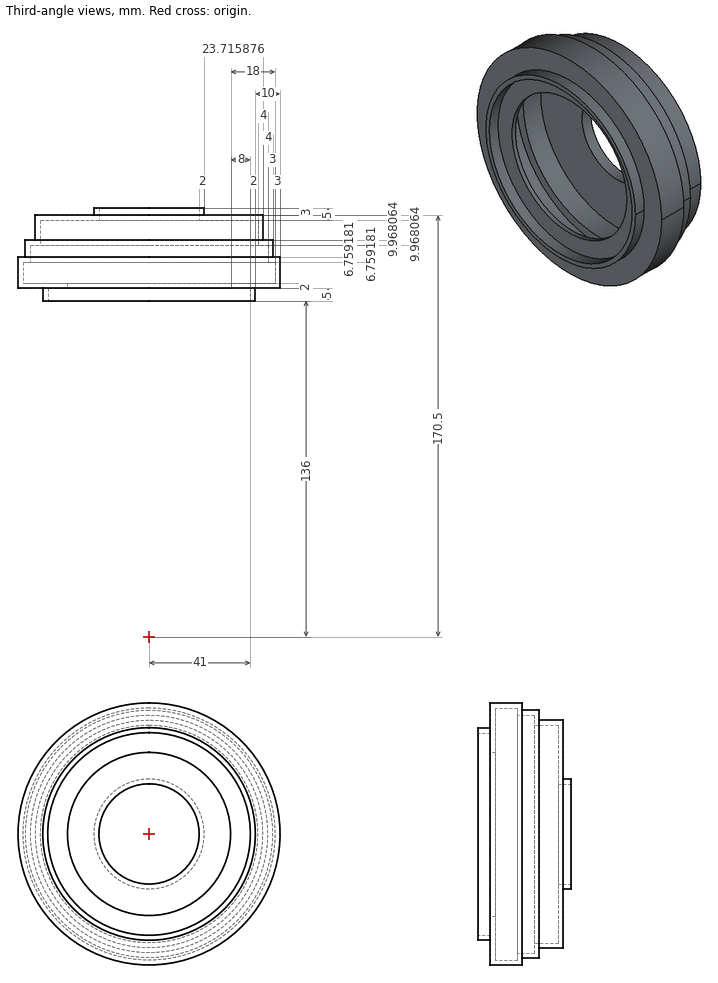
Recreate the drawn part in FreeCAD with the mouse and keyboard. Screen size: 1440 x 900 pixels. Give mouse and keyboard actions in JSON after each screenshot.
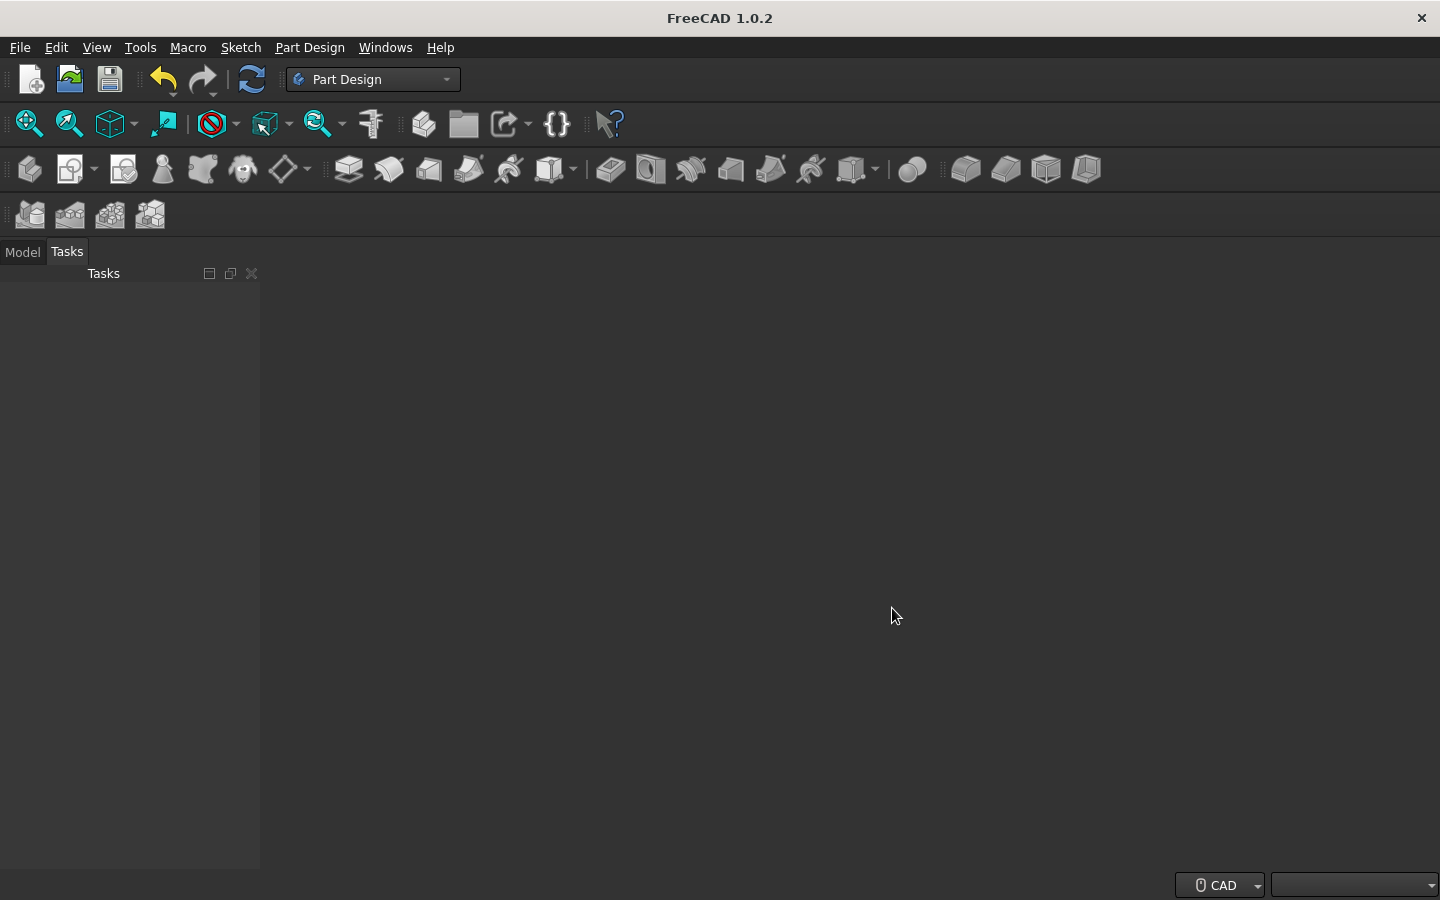
{"action": "left_click", "coordinate": [30, 80]}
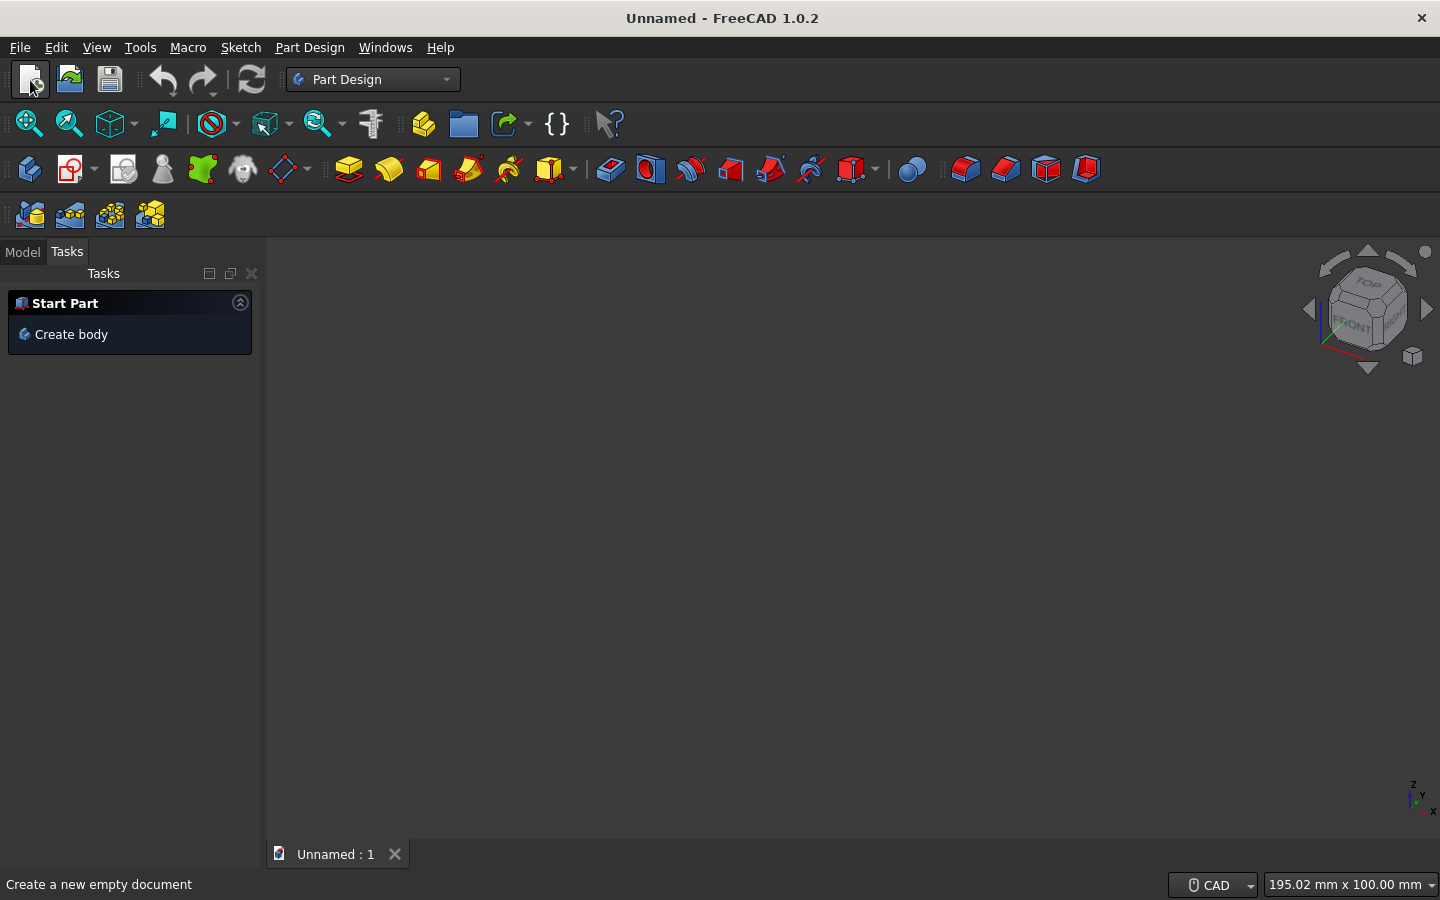
{"action": "left_click", "coordinate": [70, 170]}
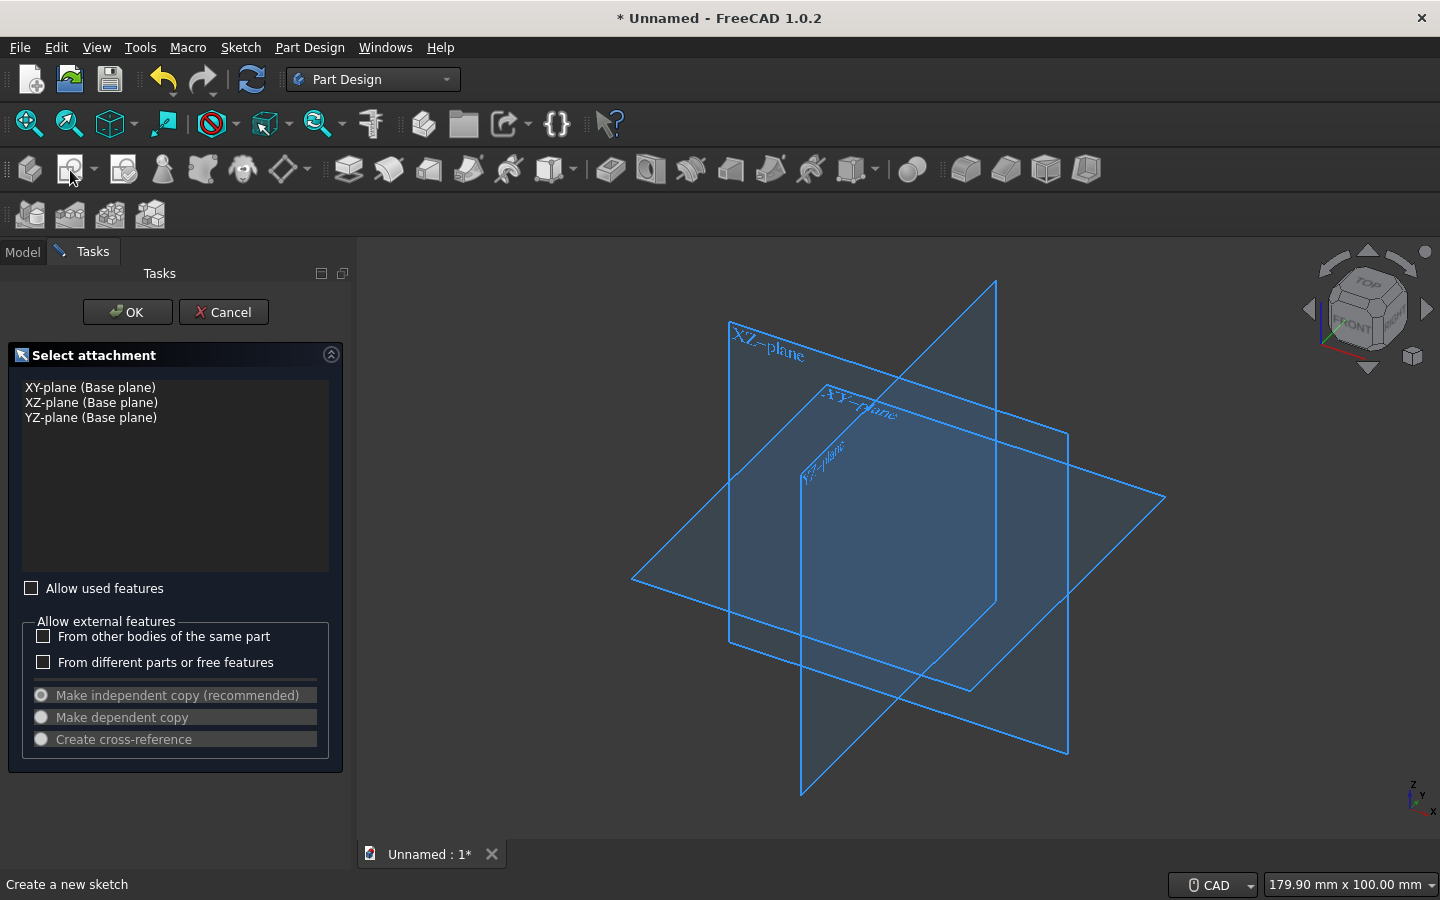
{"action": "left_click", "coordinate": [82, 388]}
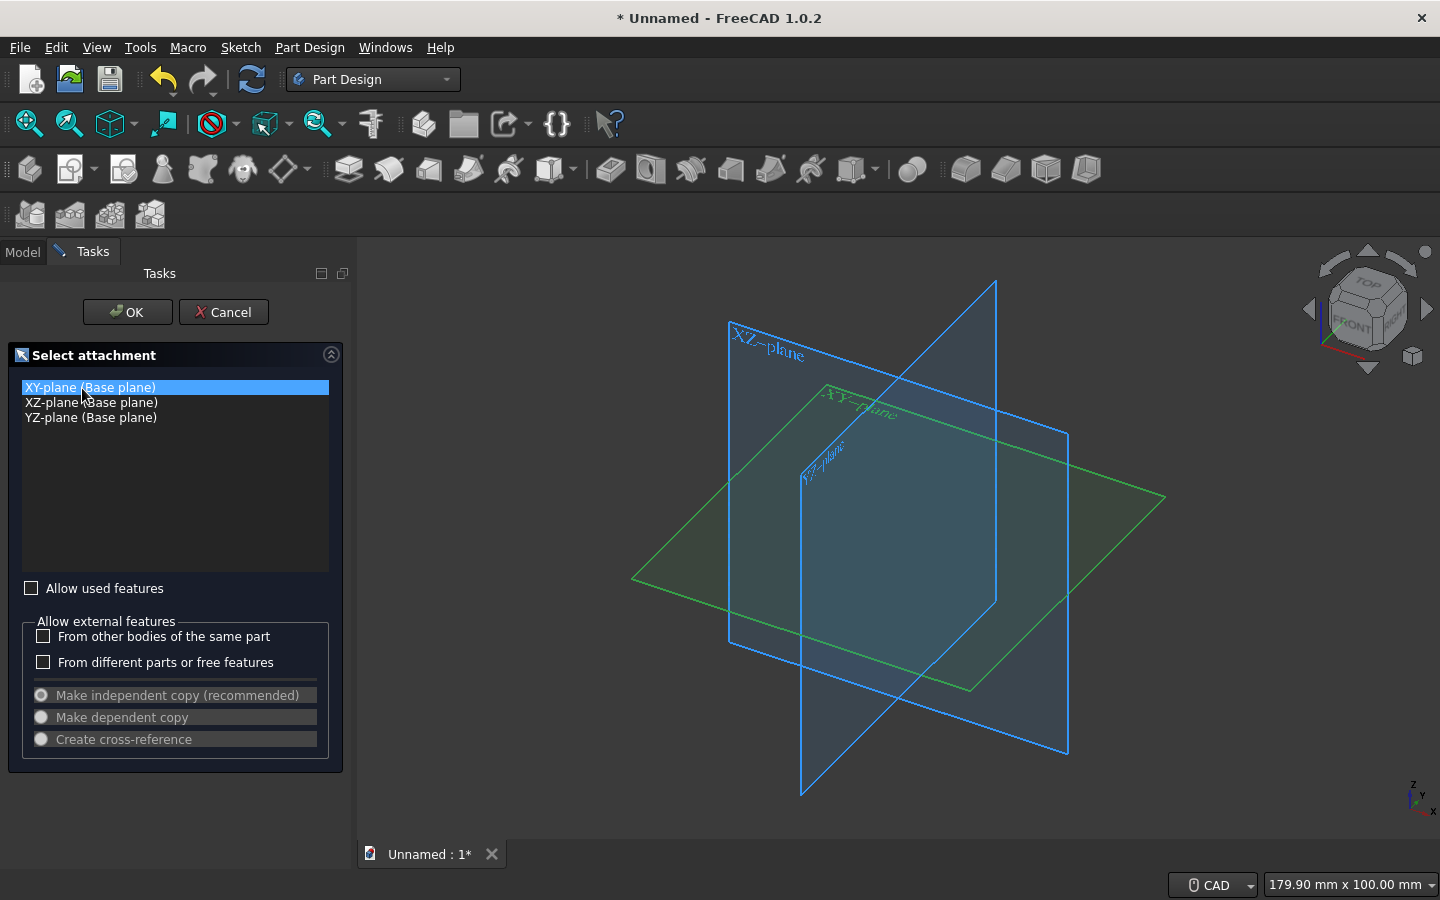
{"action": "left_click", "coordinate": [128, 312]}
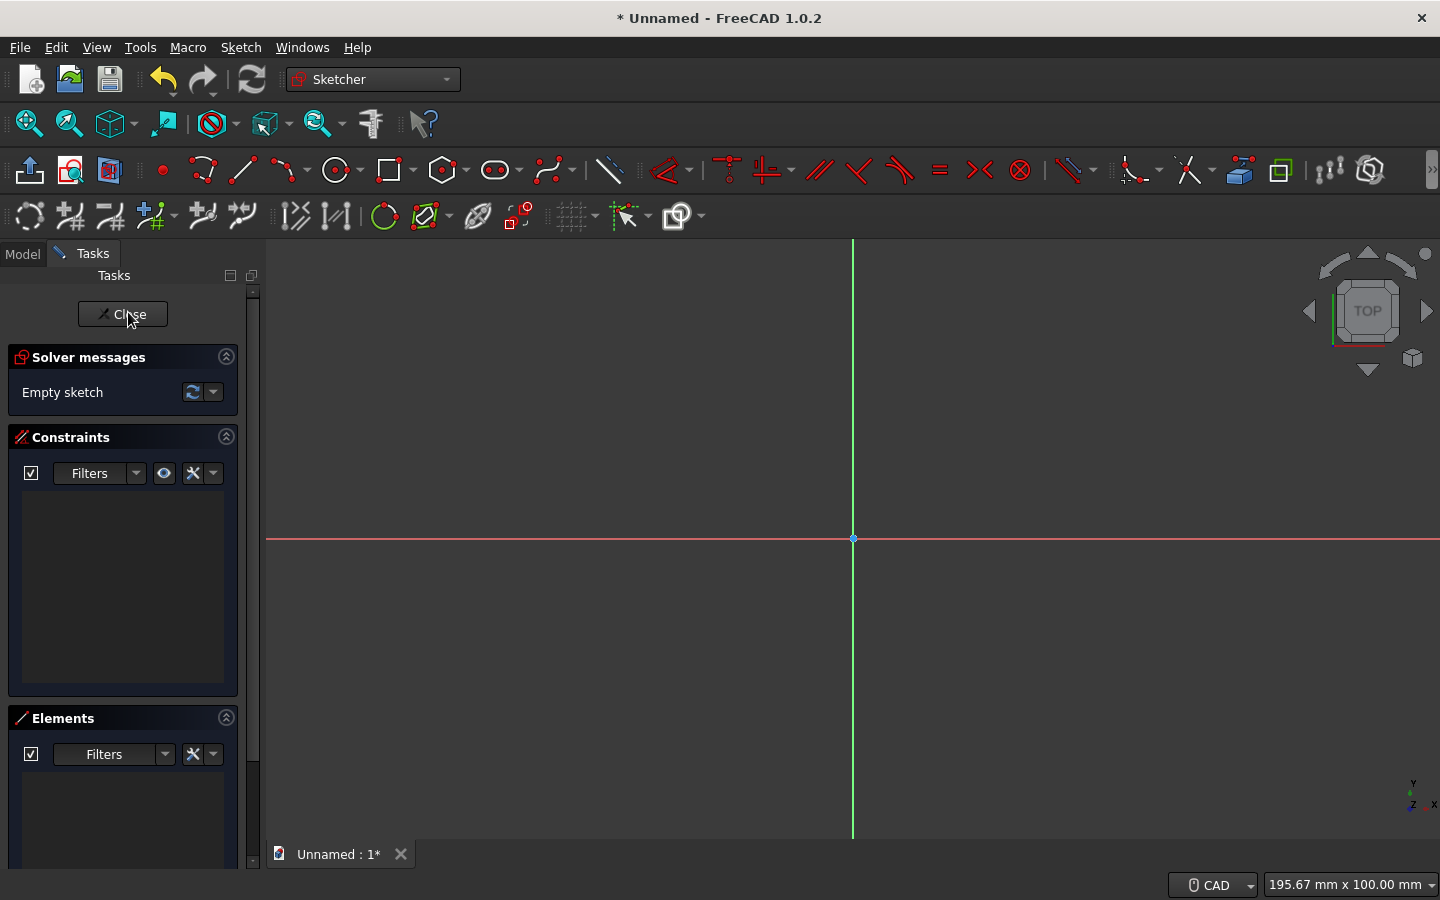
{"action": "scroll", "coordinate": [784, 539], "scroll_direction": "down", "scroll_amount": 5}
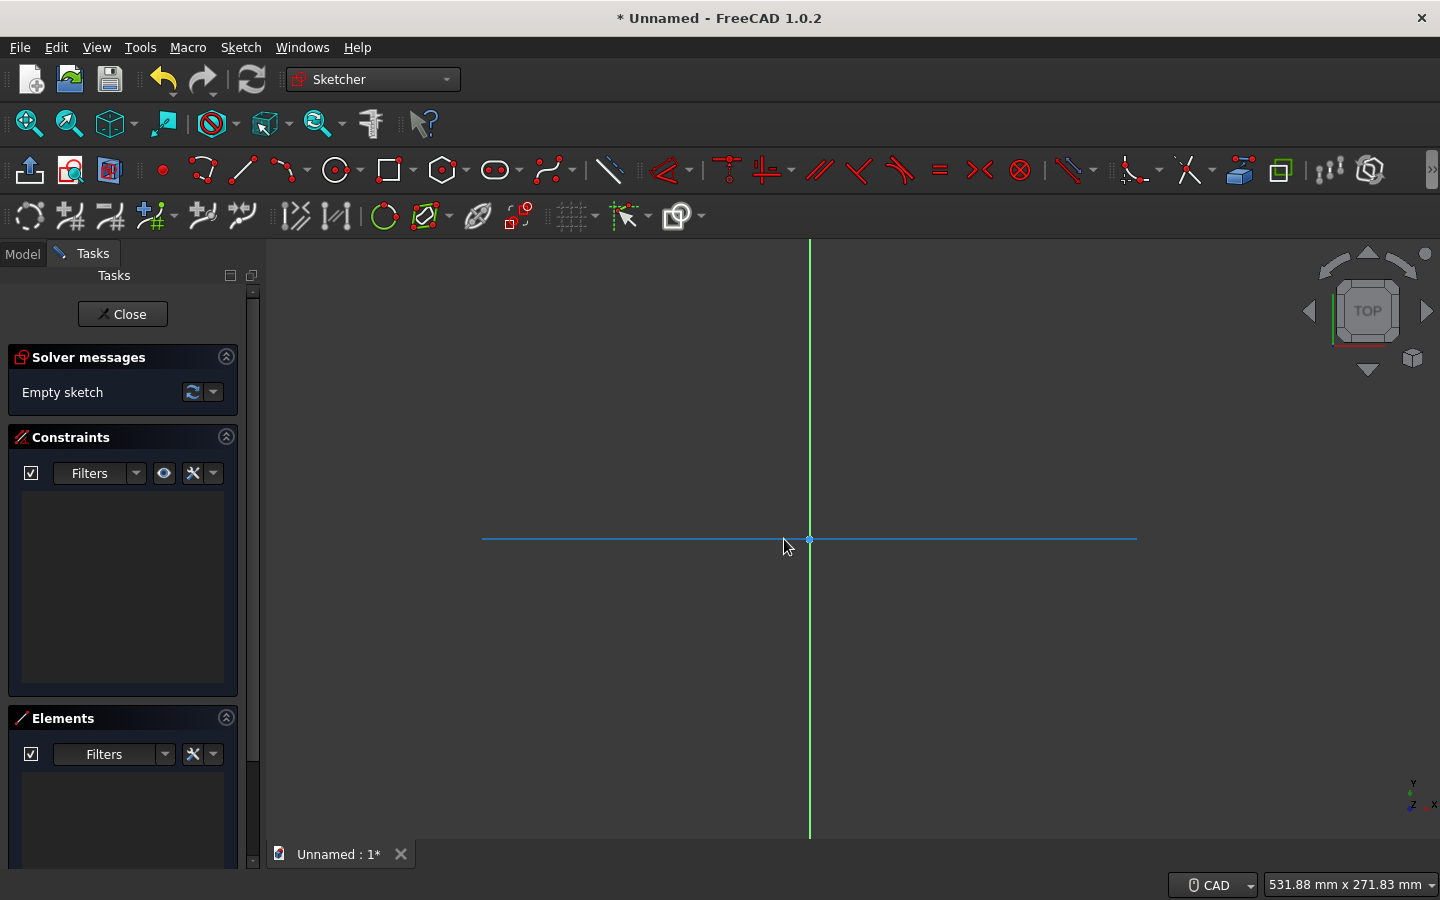
{"action": "scroll", "coordinate": [784, 539], "scroll_direction": "down", "scroll_amount": 5}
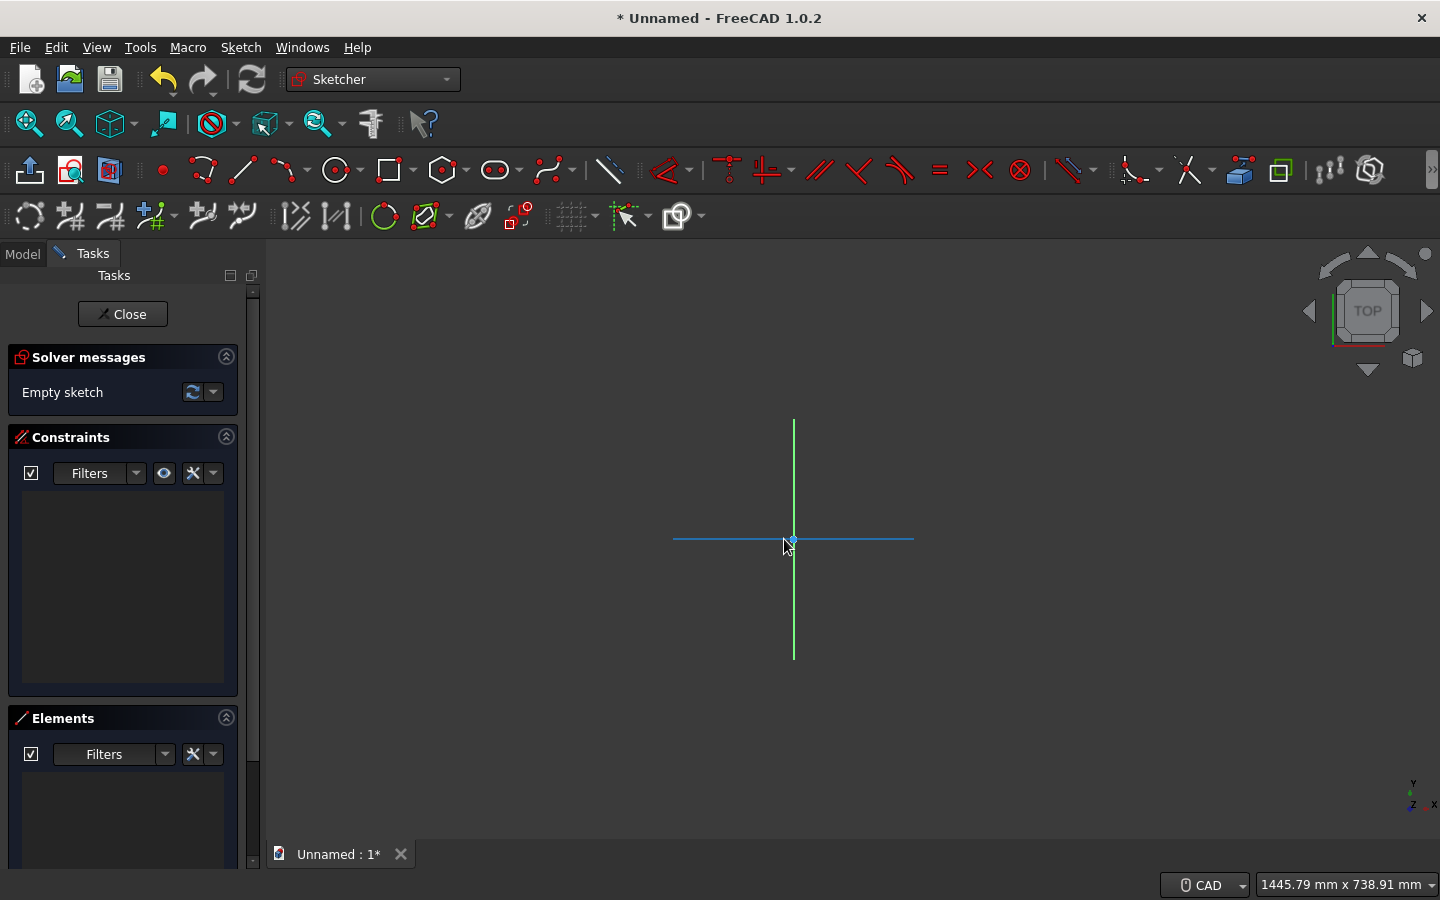
{"action": "scroll", "coordinate": [827, 404], "scroll_direction": "up", "scroll_amount": 13}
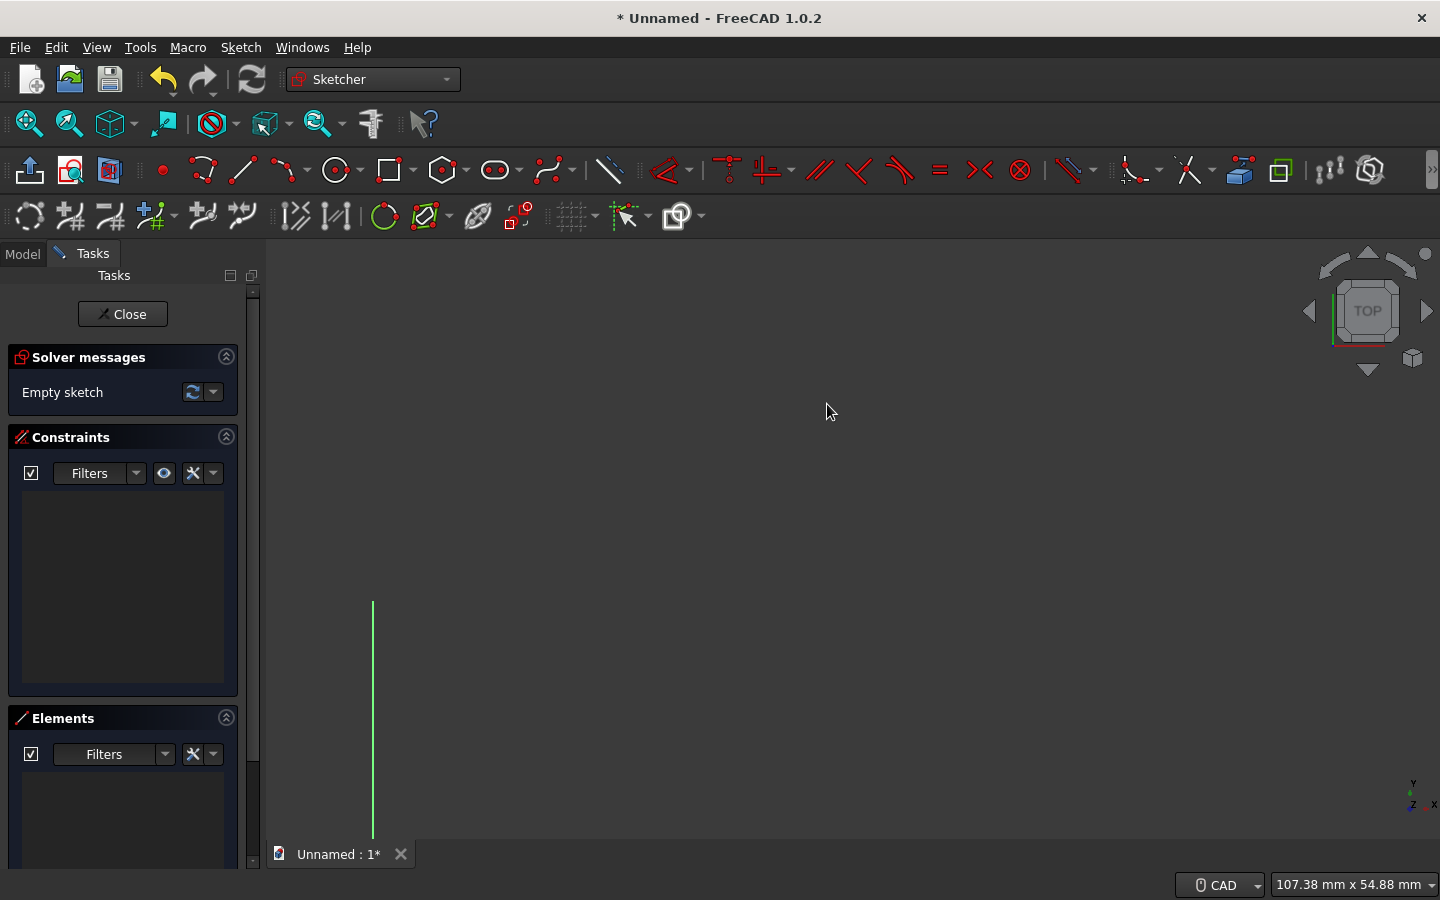
{"action": "left_click", "coordinate": [204, 170]}